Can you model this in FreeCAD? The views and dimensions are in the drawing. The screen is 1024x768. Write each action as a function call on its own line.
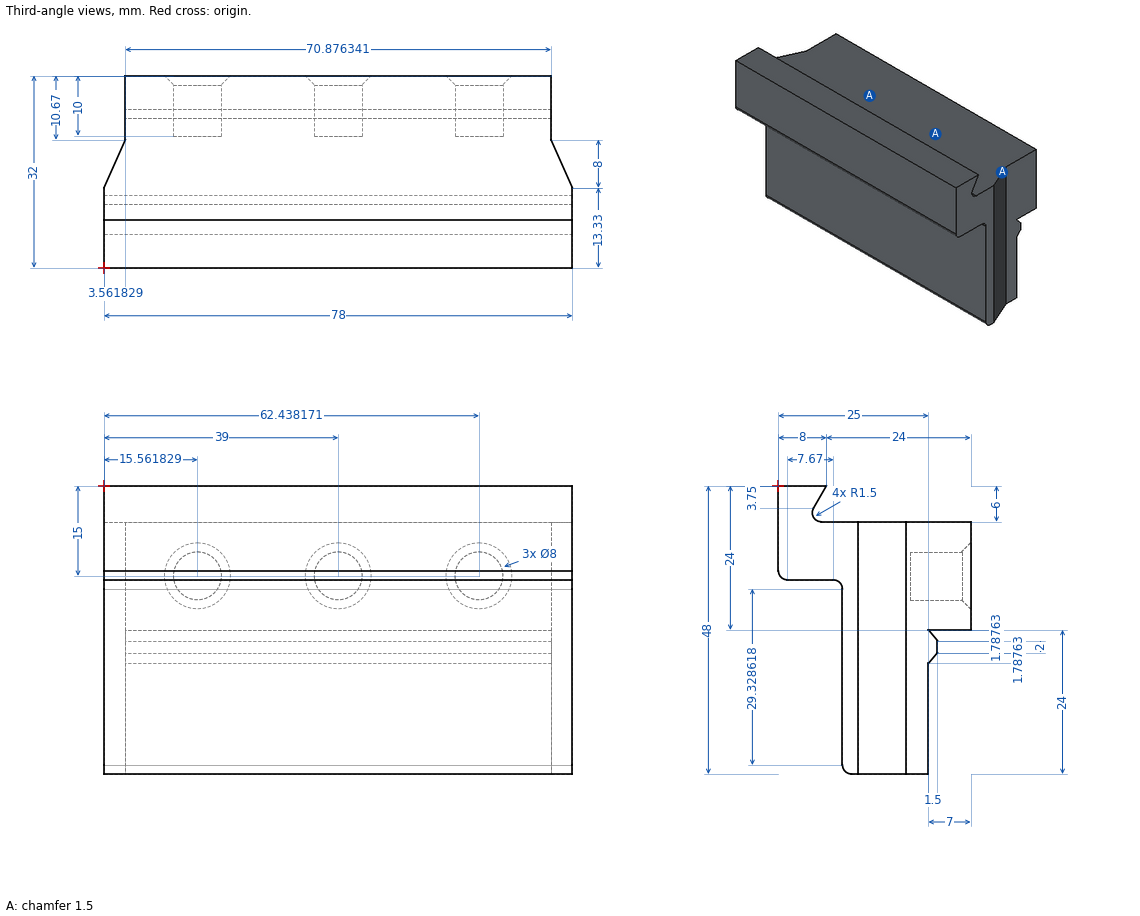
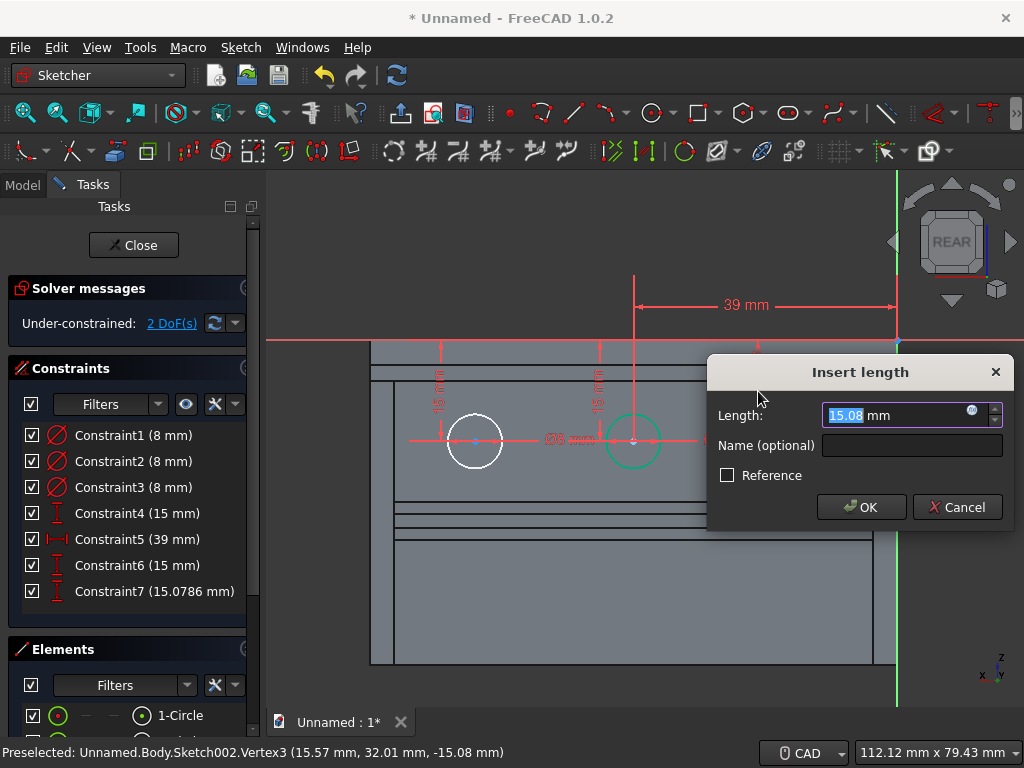
text(15)
key(Return)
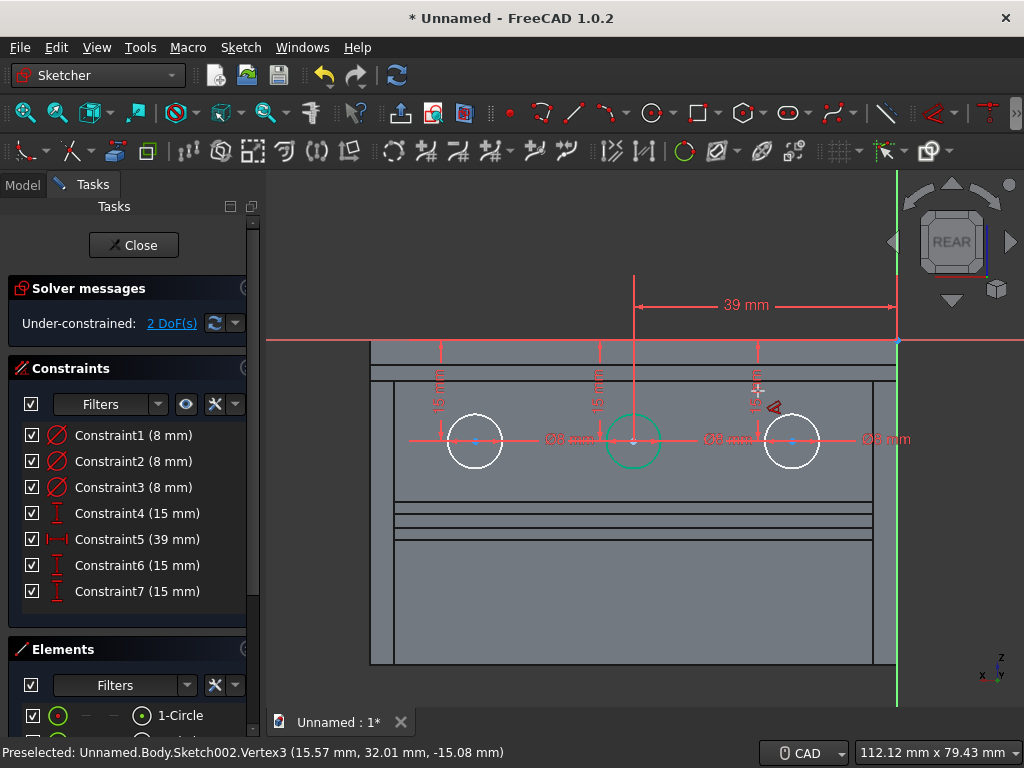
click(475, 441)
click(667, 306)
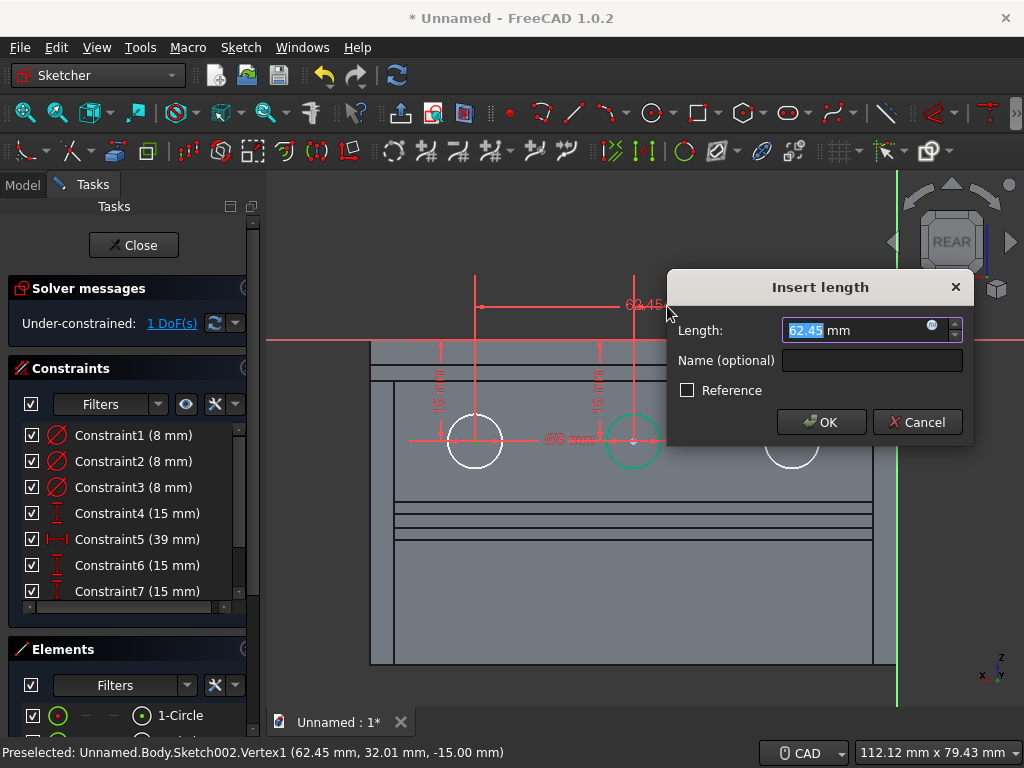
text(62.438171)
key(Return)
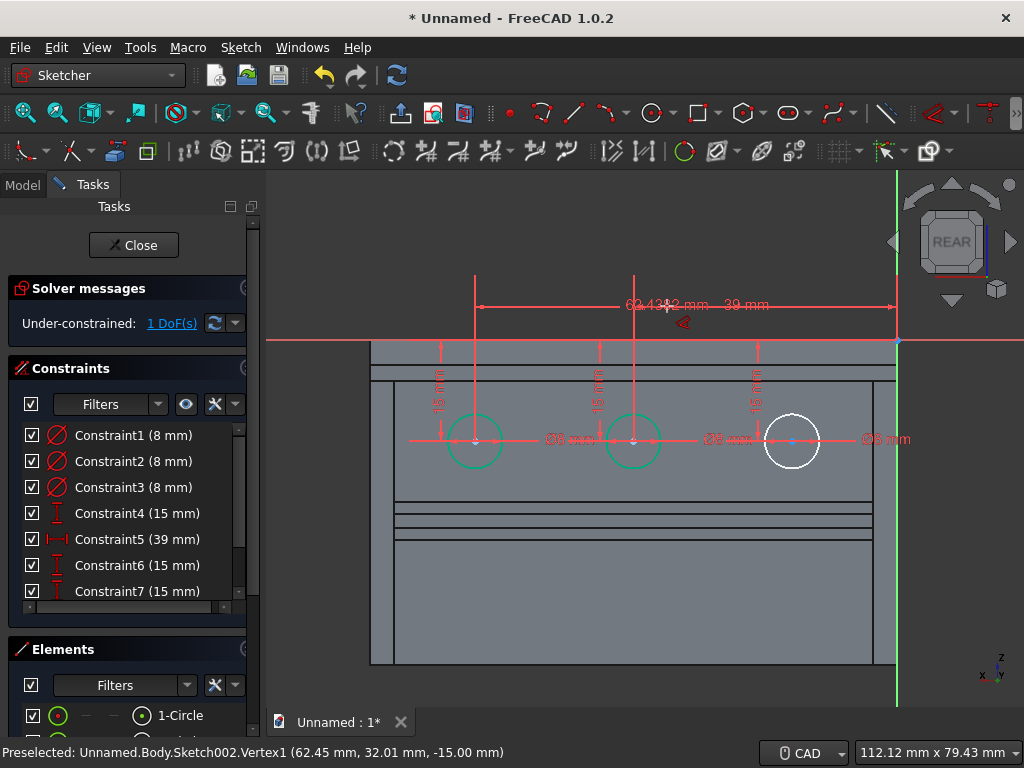
click(792, 441)
click(826, 306)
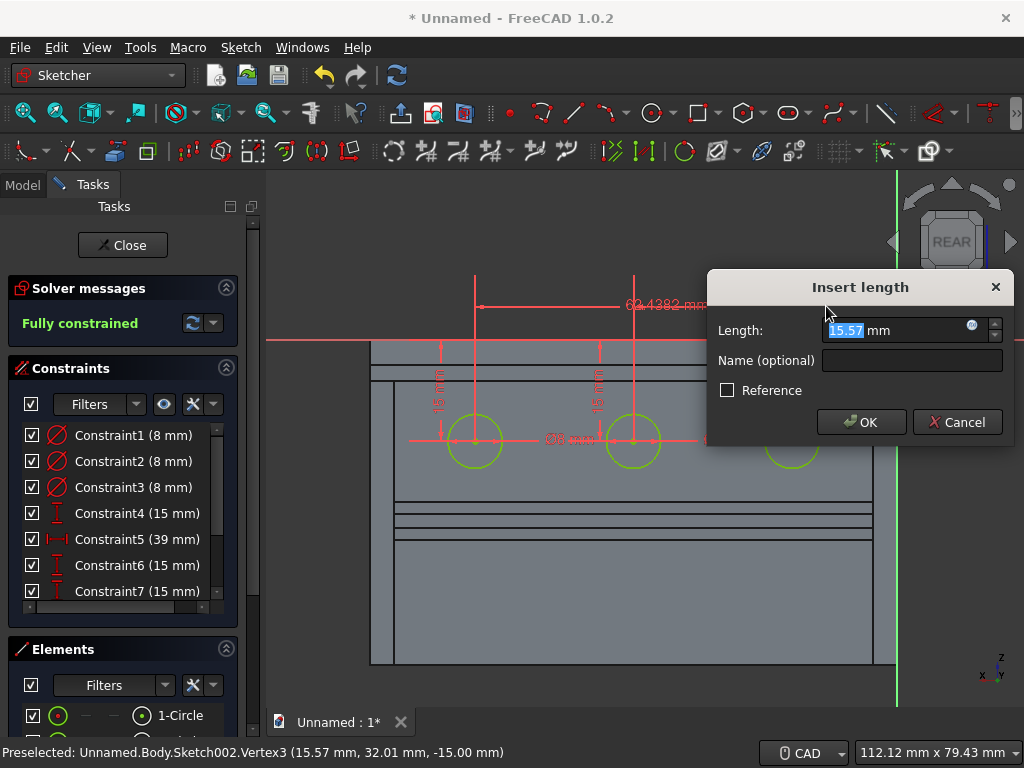
text(15.561829)
key(Return)
key(Escape)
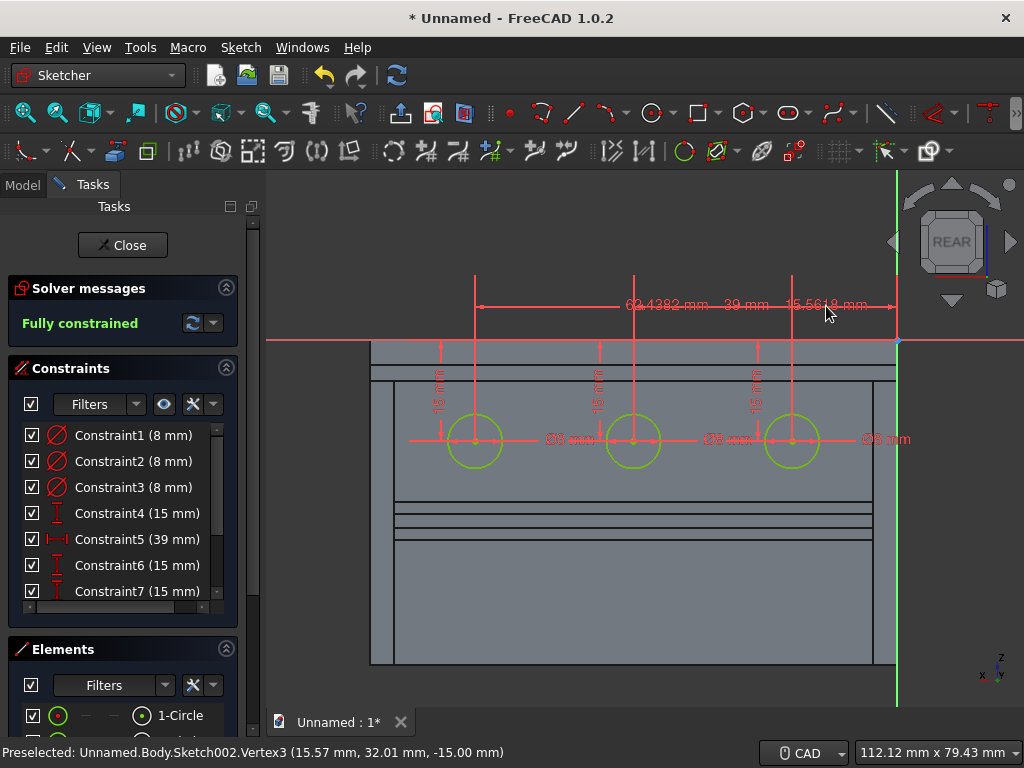
click(123, 245)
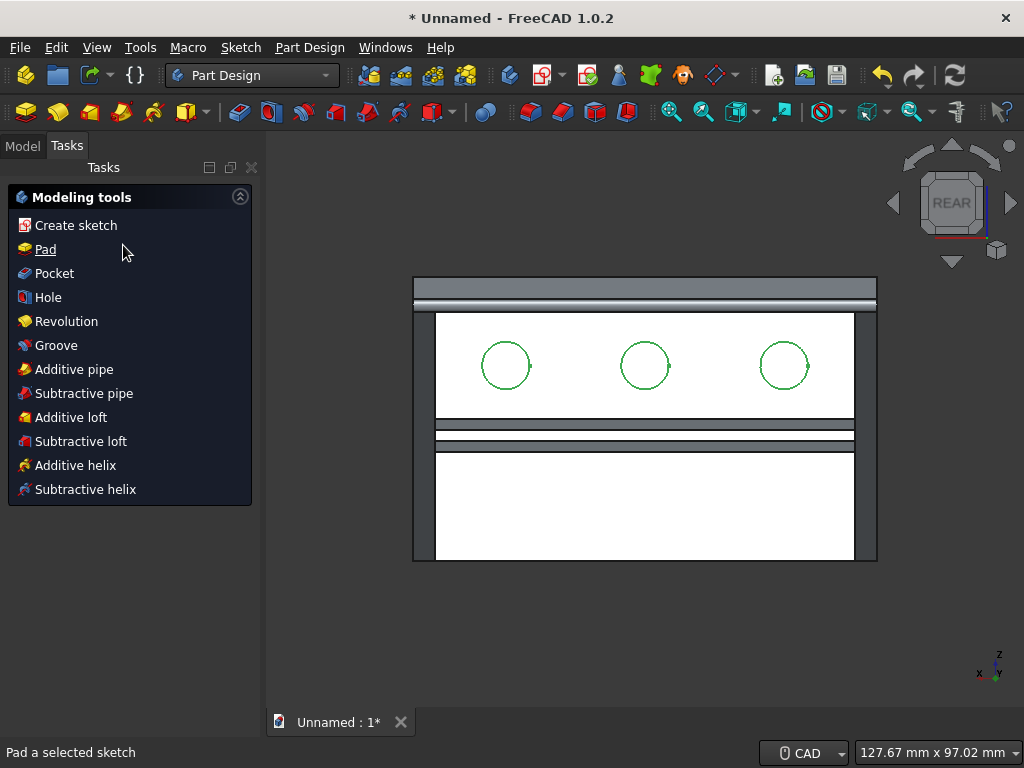
click(240, 112)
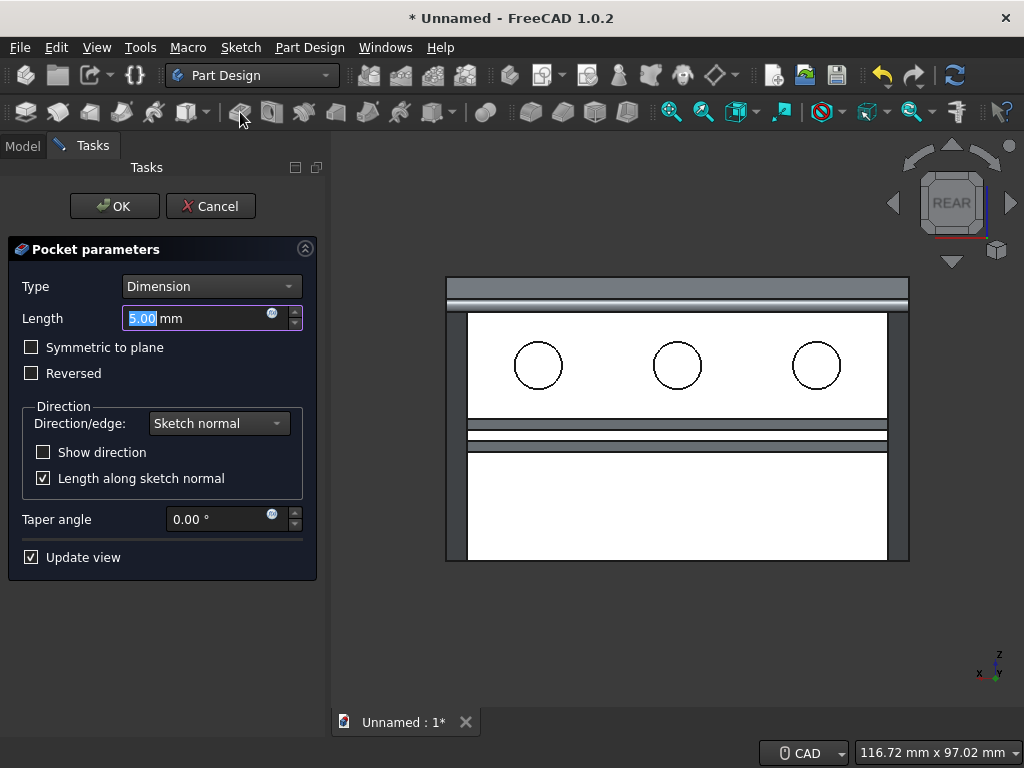
text(10)
key(Tab)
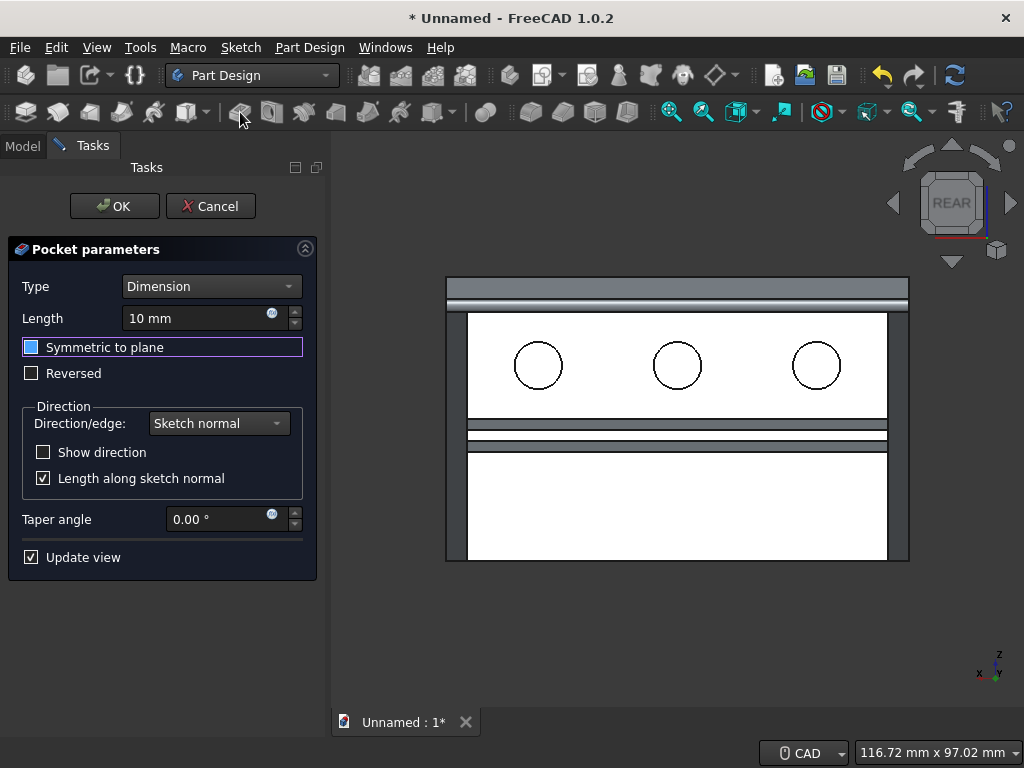
click(115, 206)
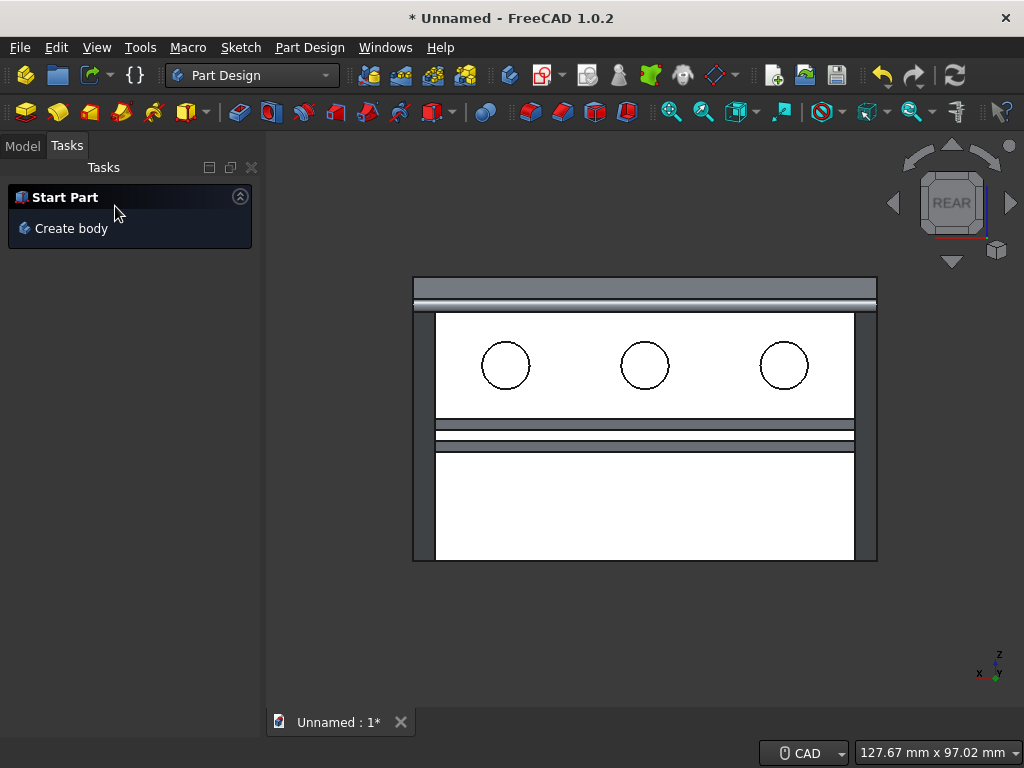
click(482, 365)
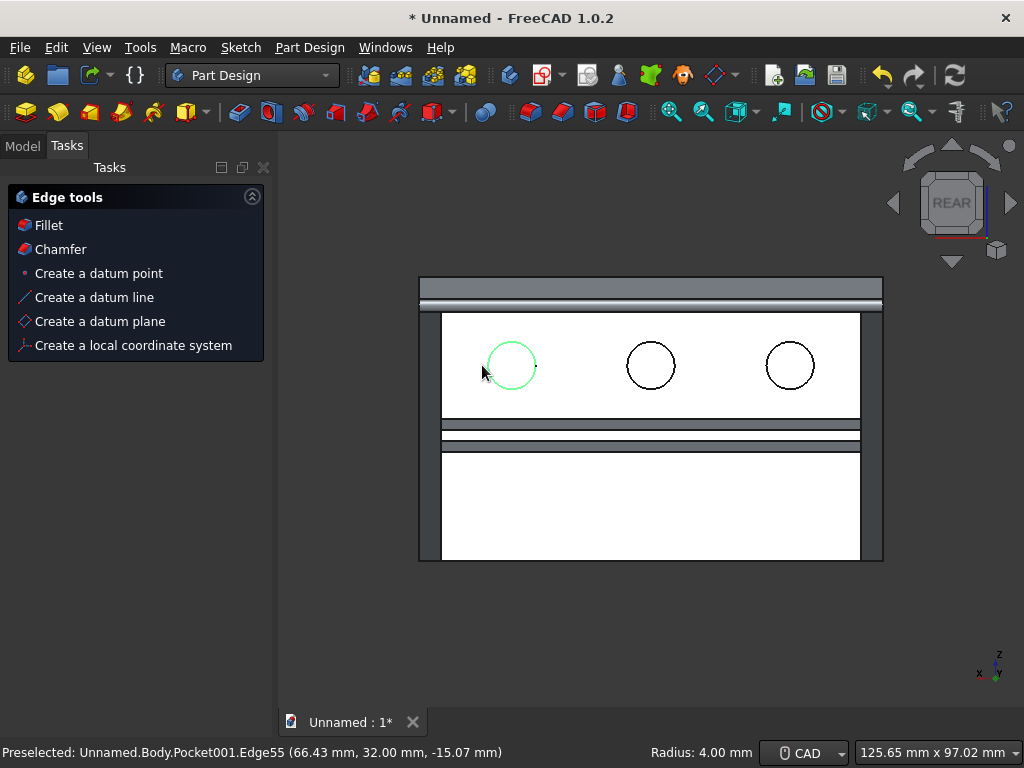
click(627, 365, ctrl)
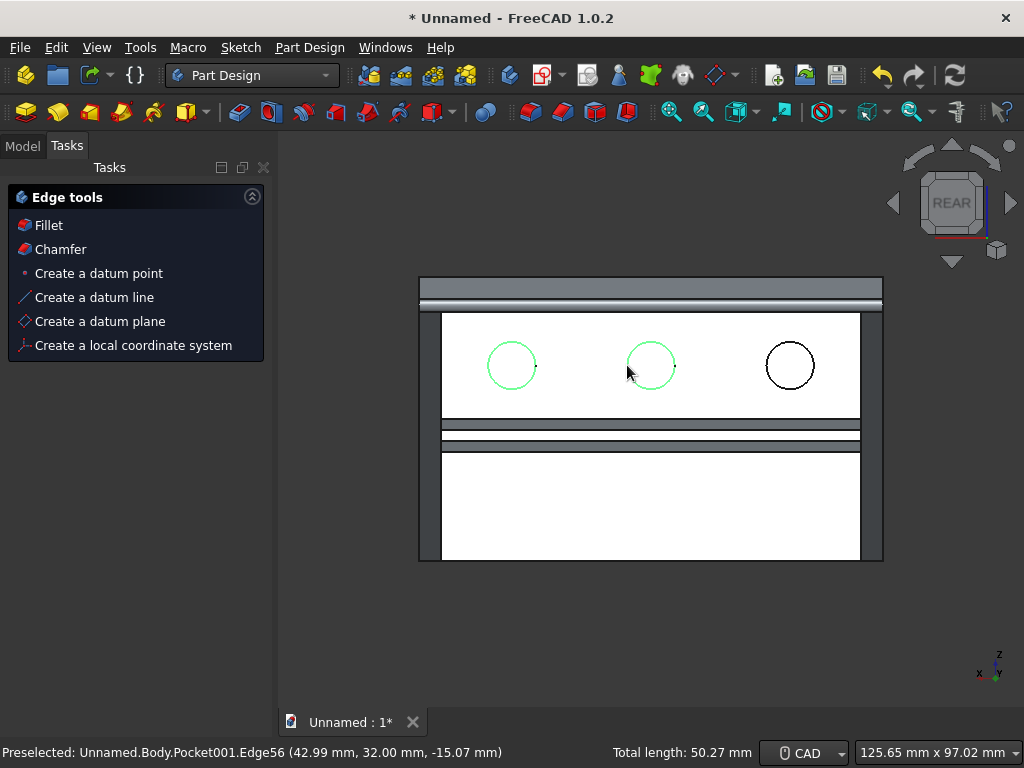
click(766, 365, ctrl)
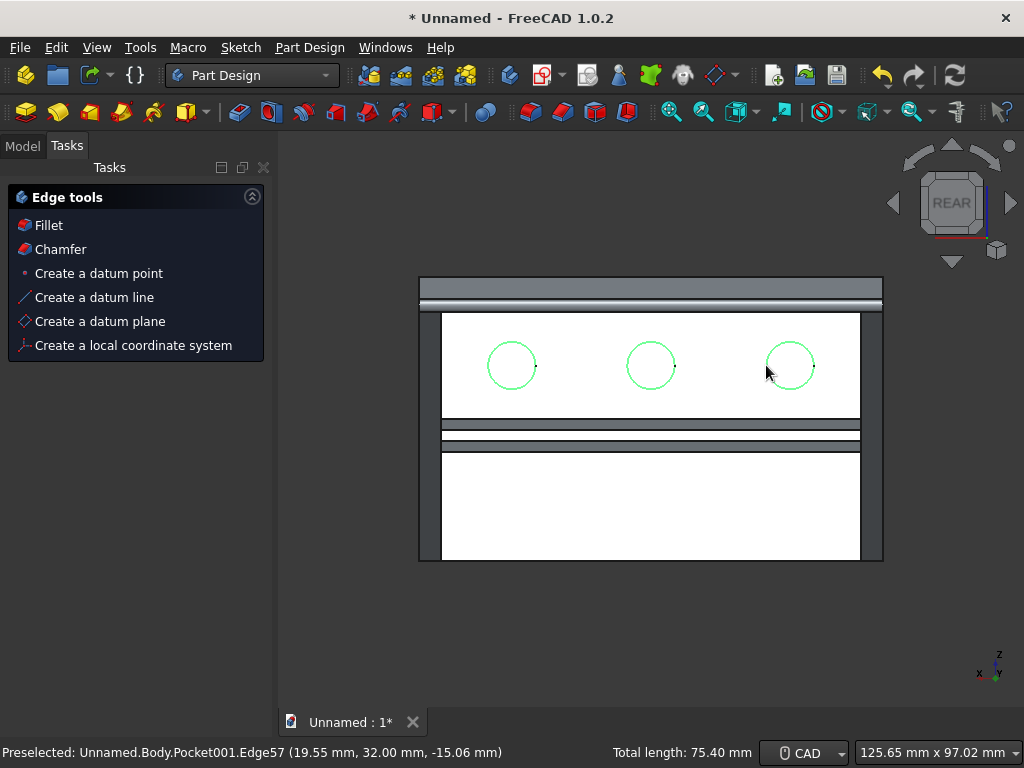
click(564, 112)